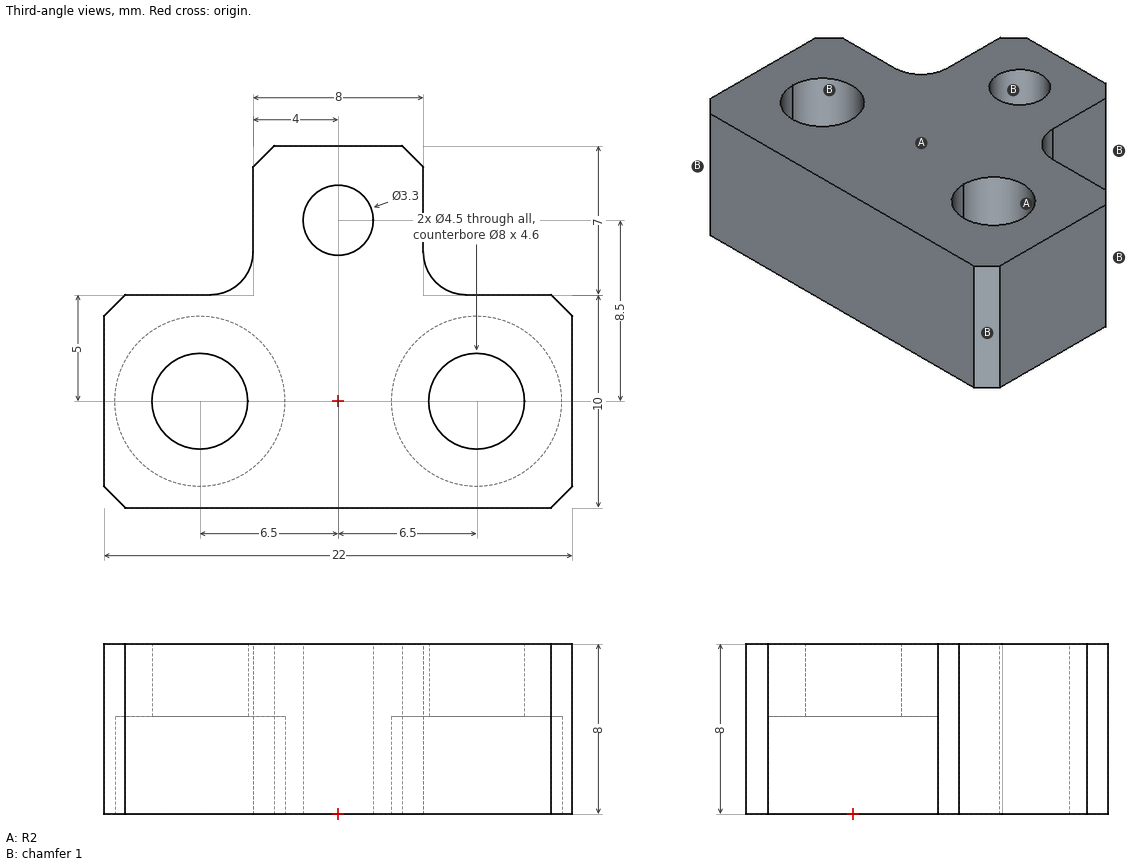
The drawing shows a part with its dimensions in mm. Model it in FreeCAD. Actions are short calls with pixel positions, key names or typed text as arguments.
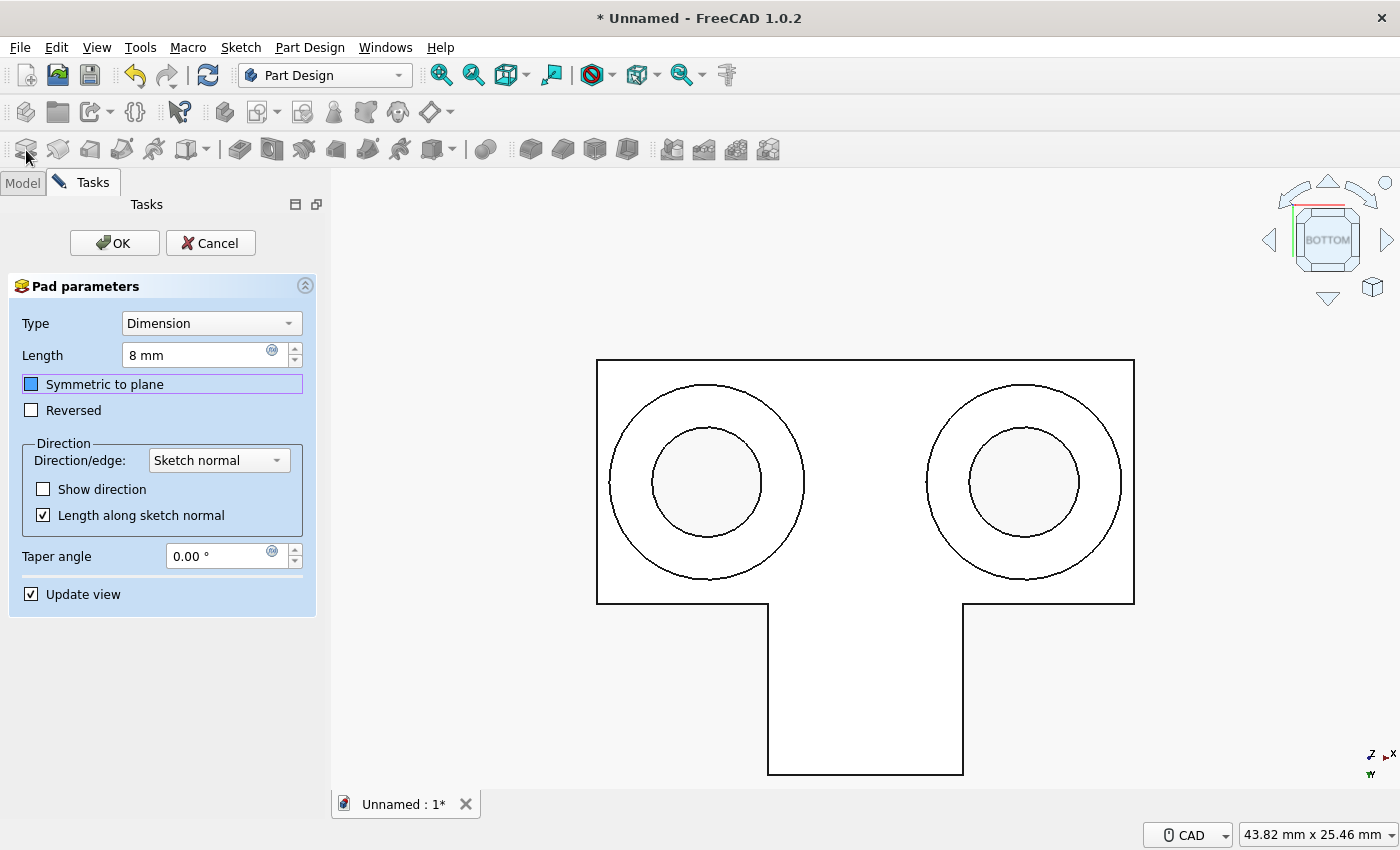
click(115, 243)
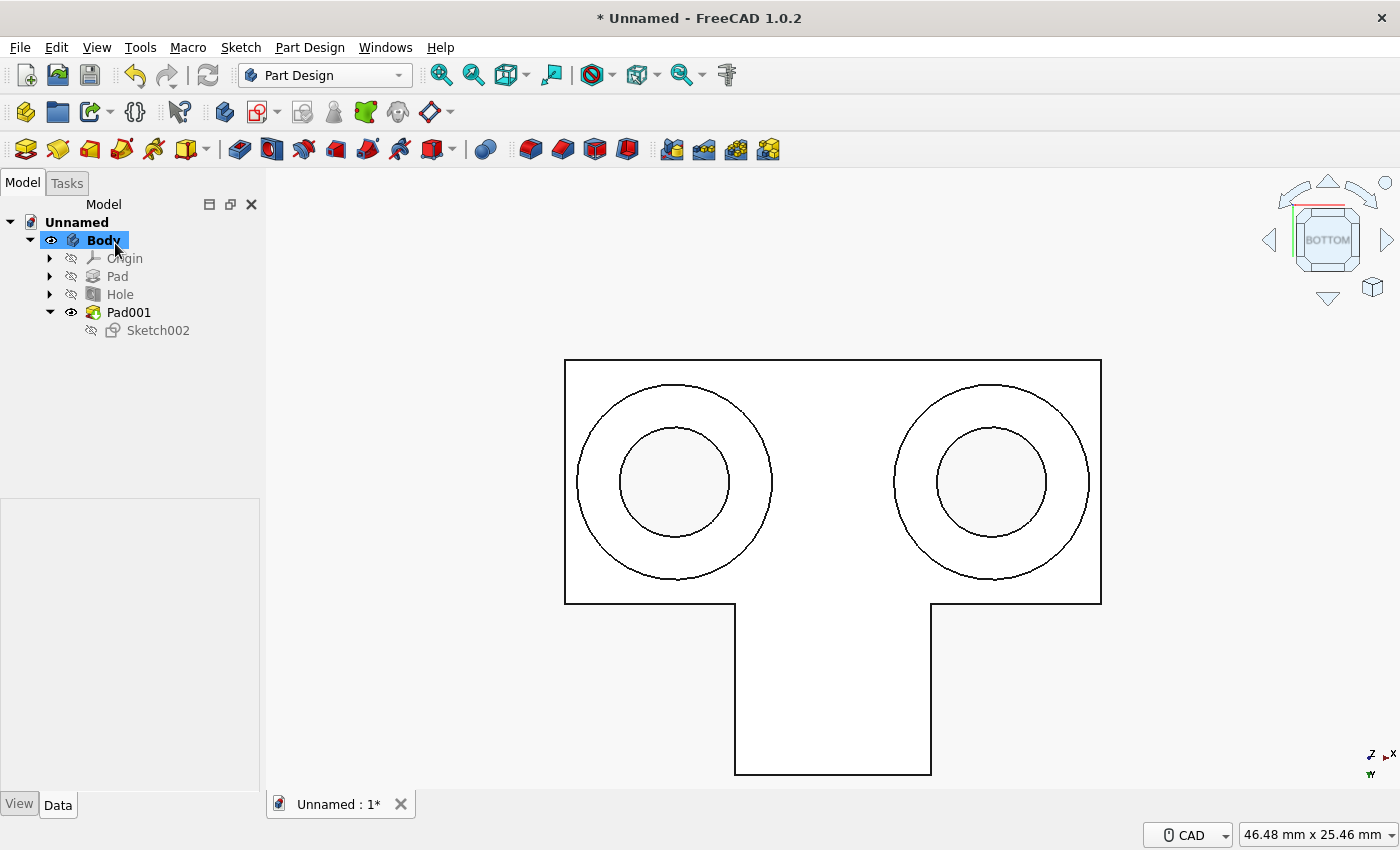
click(833, 626)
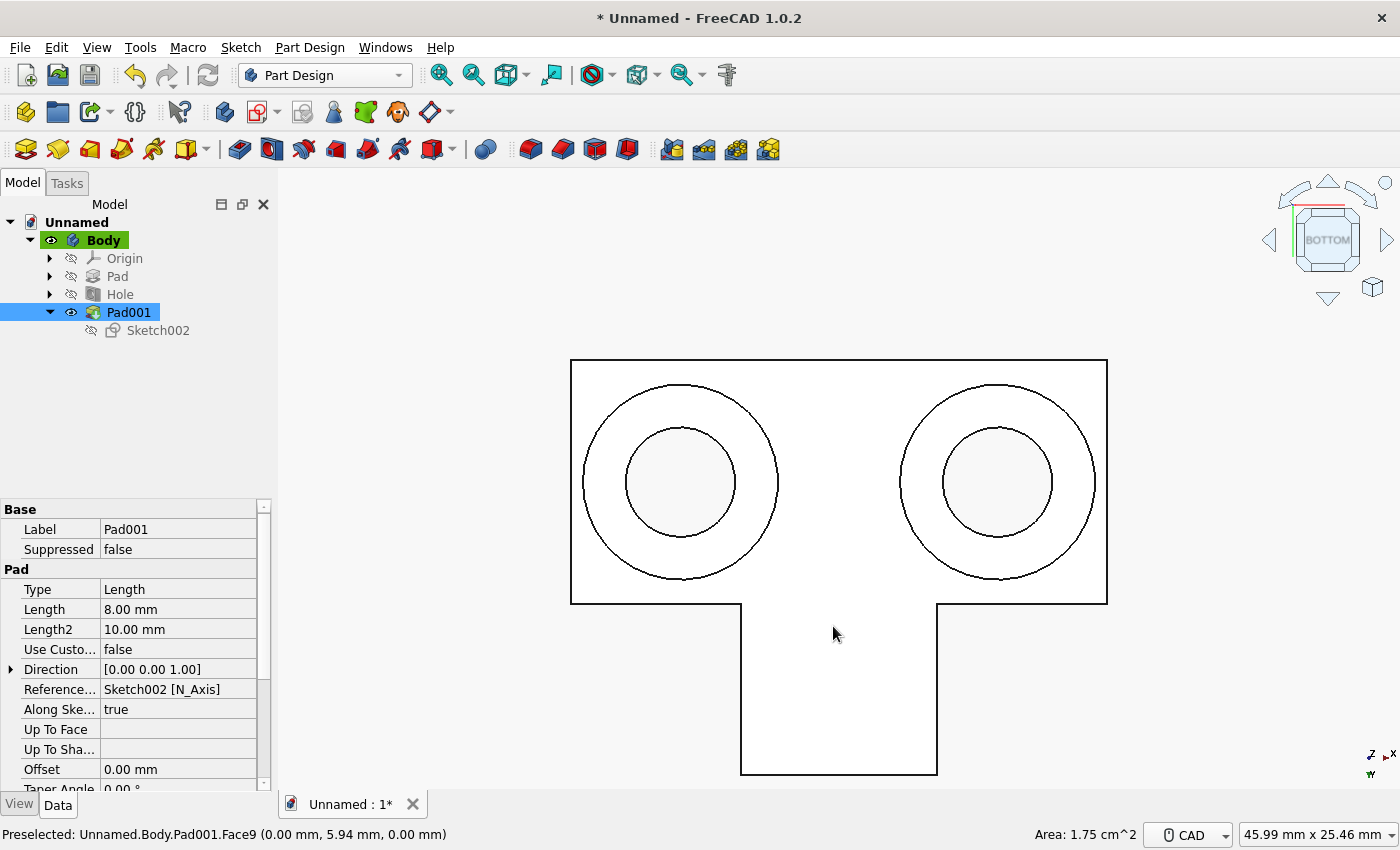
click(258, 112)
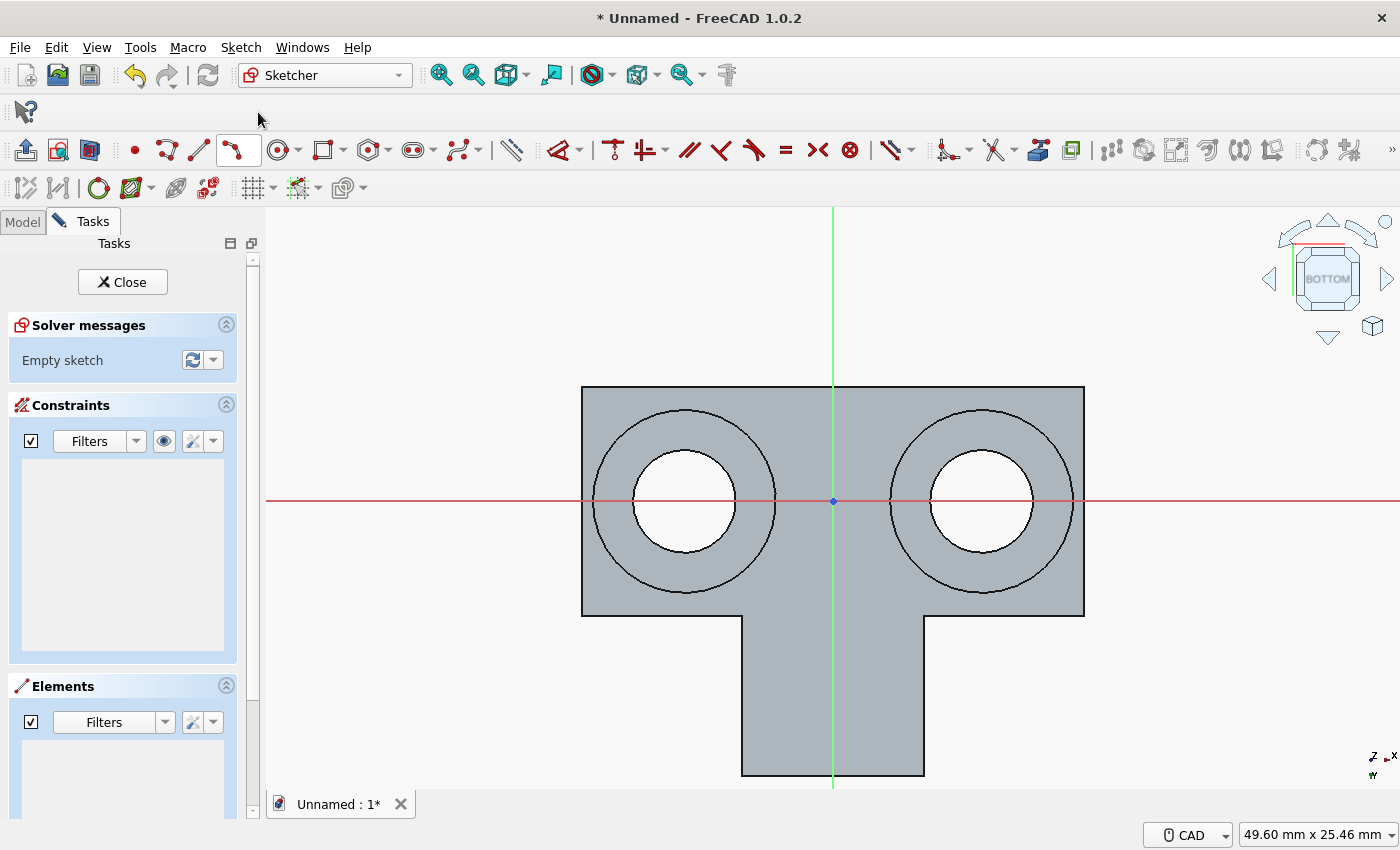
scroll(850, 746, up, 8)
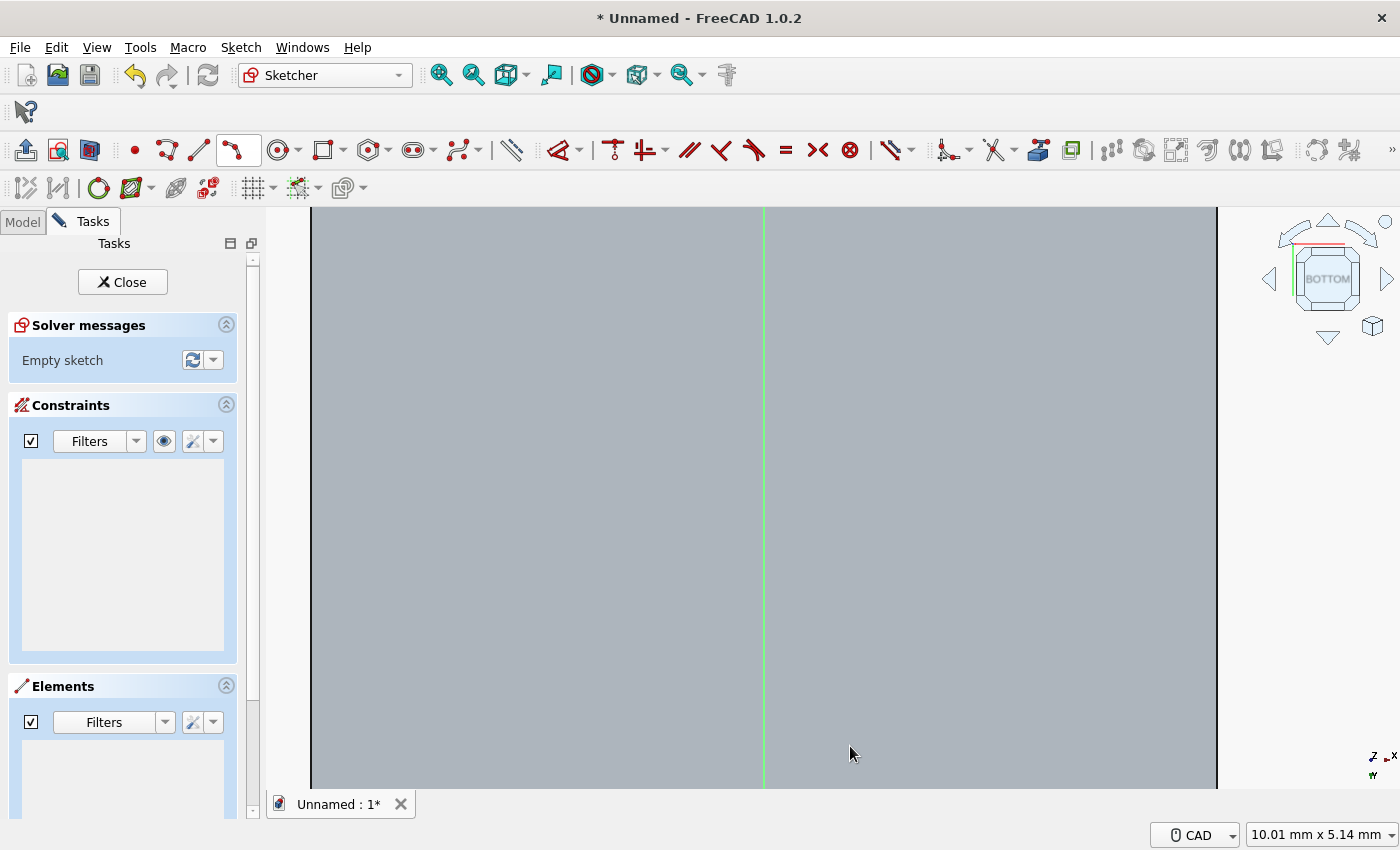
click(278, 150)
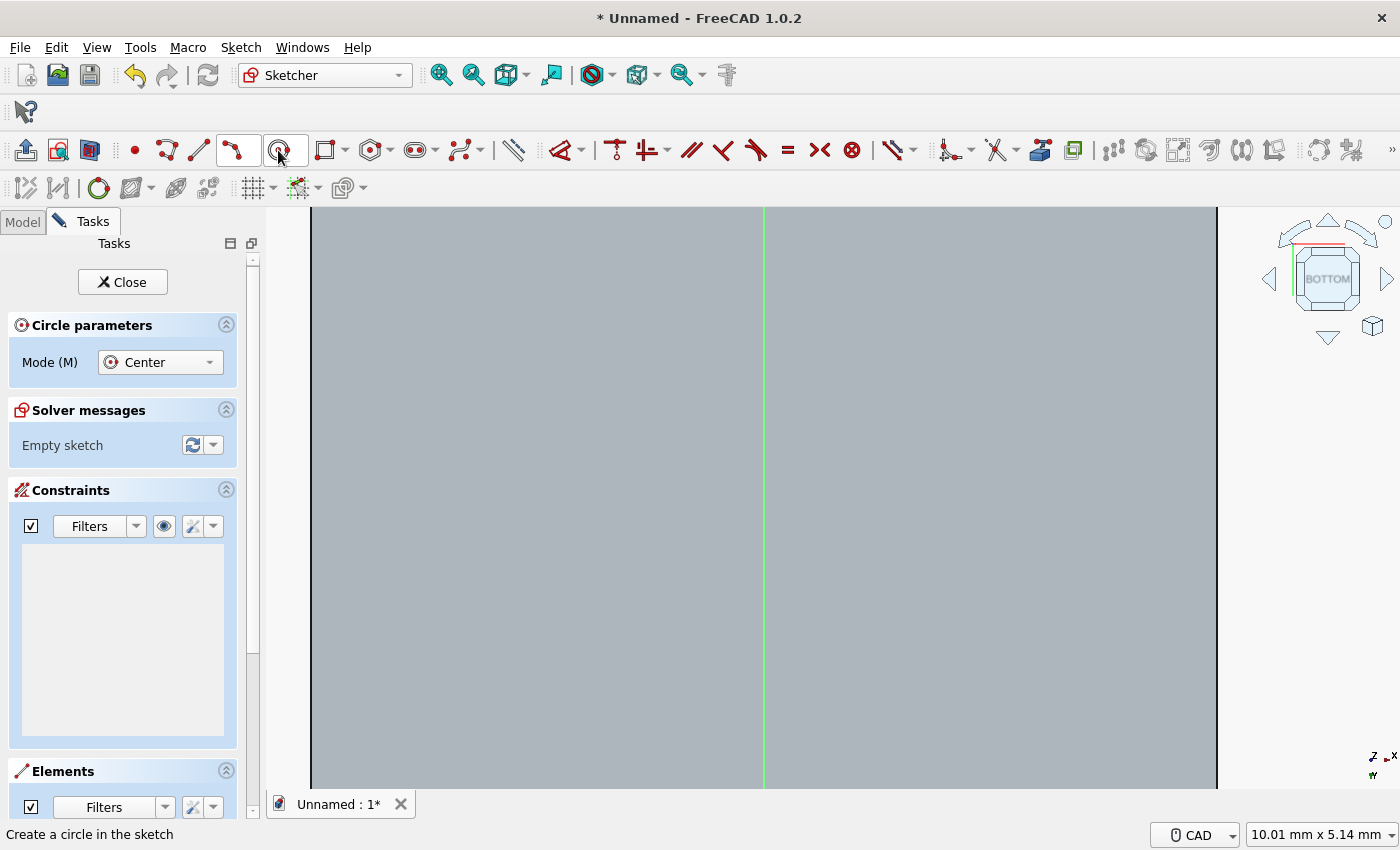
click(764, 493)
move(896, 361)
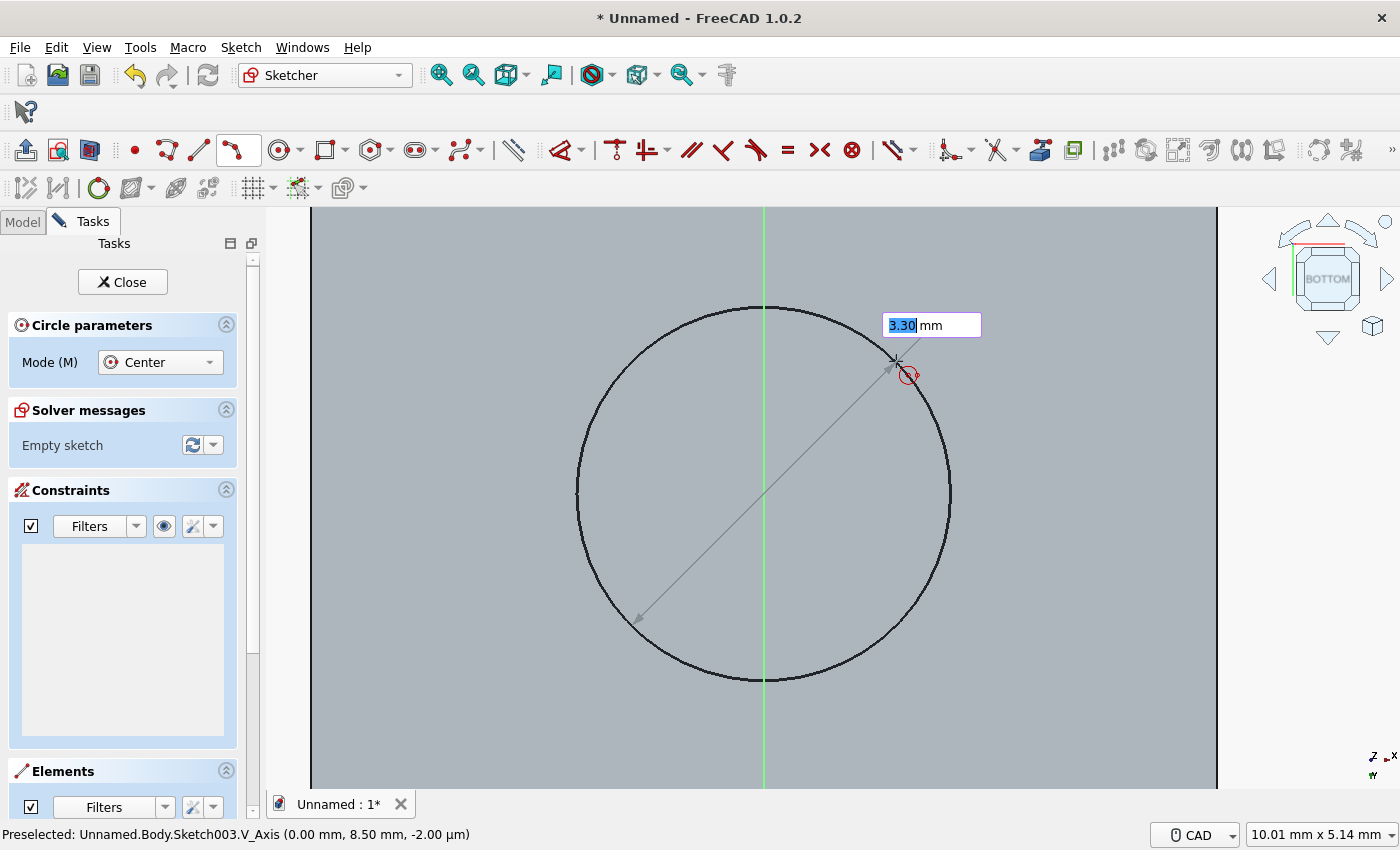
text(3.3)
key(Return)
key(Escape)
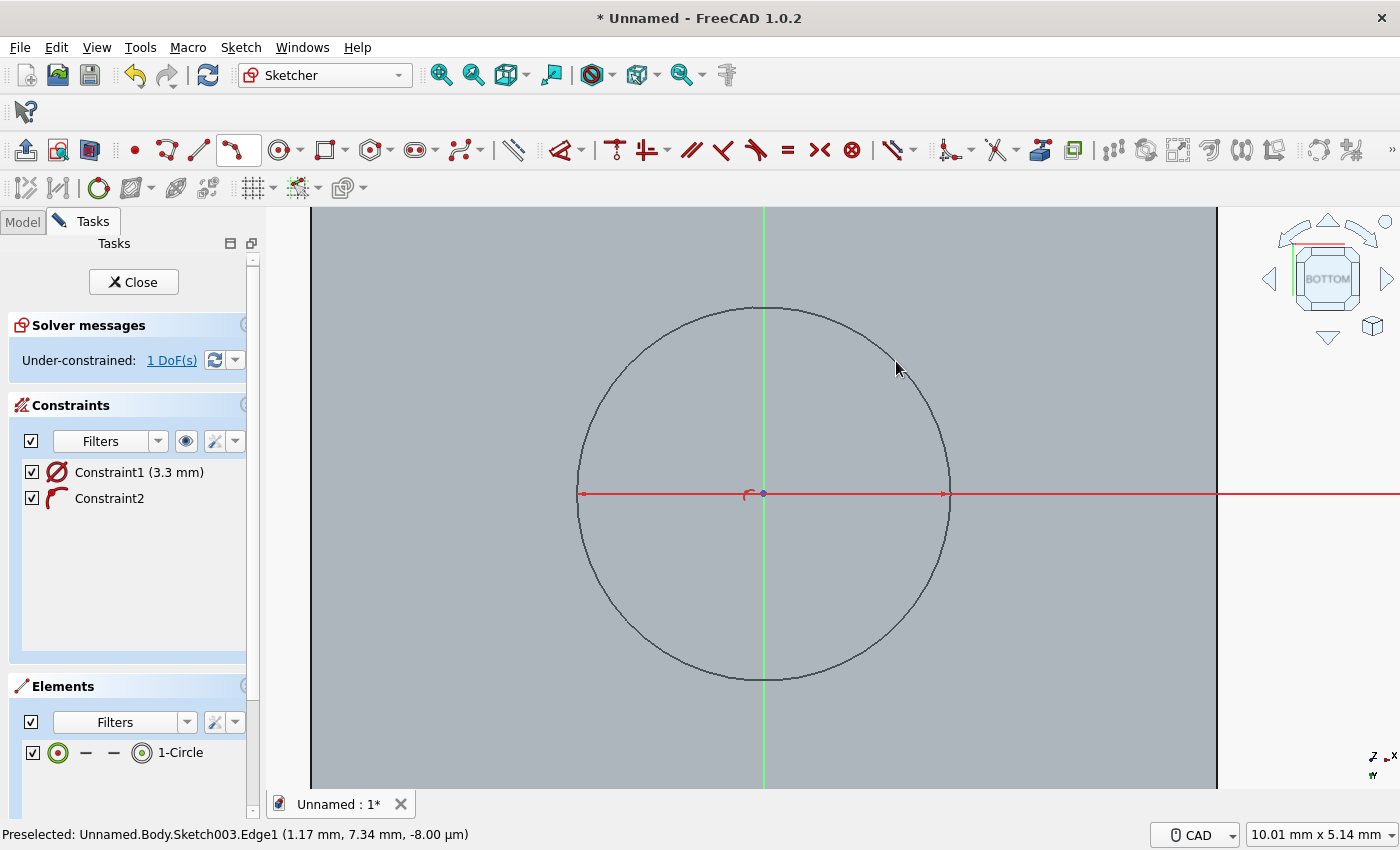
click(560, 150)